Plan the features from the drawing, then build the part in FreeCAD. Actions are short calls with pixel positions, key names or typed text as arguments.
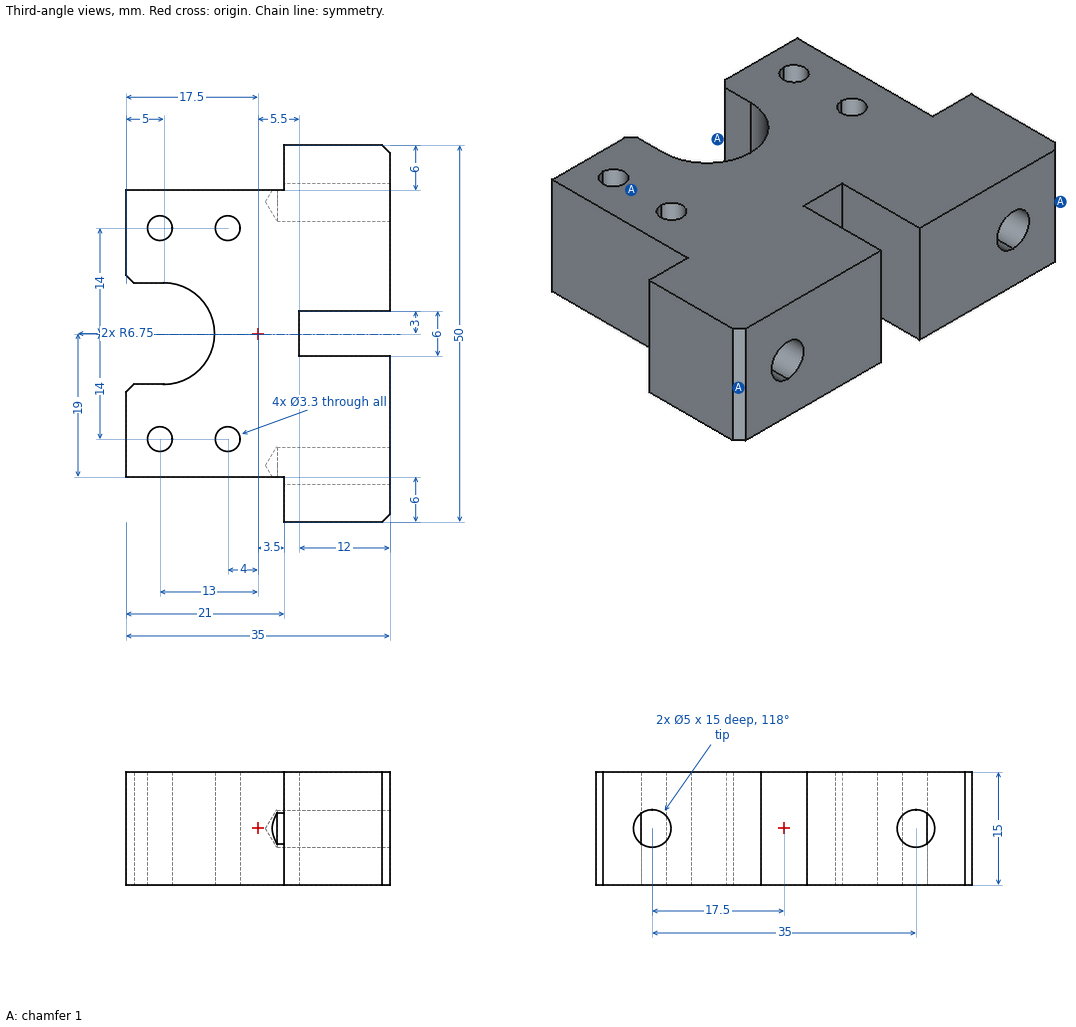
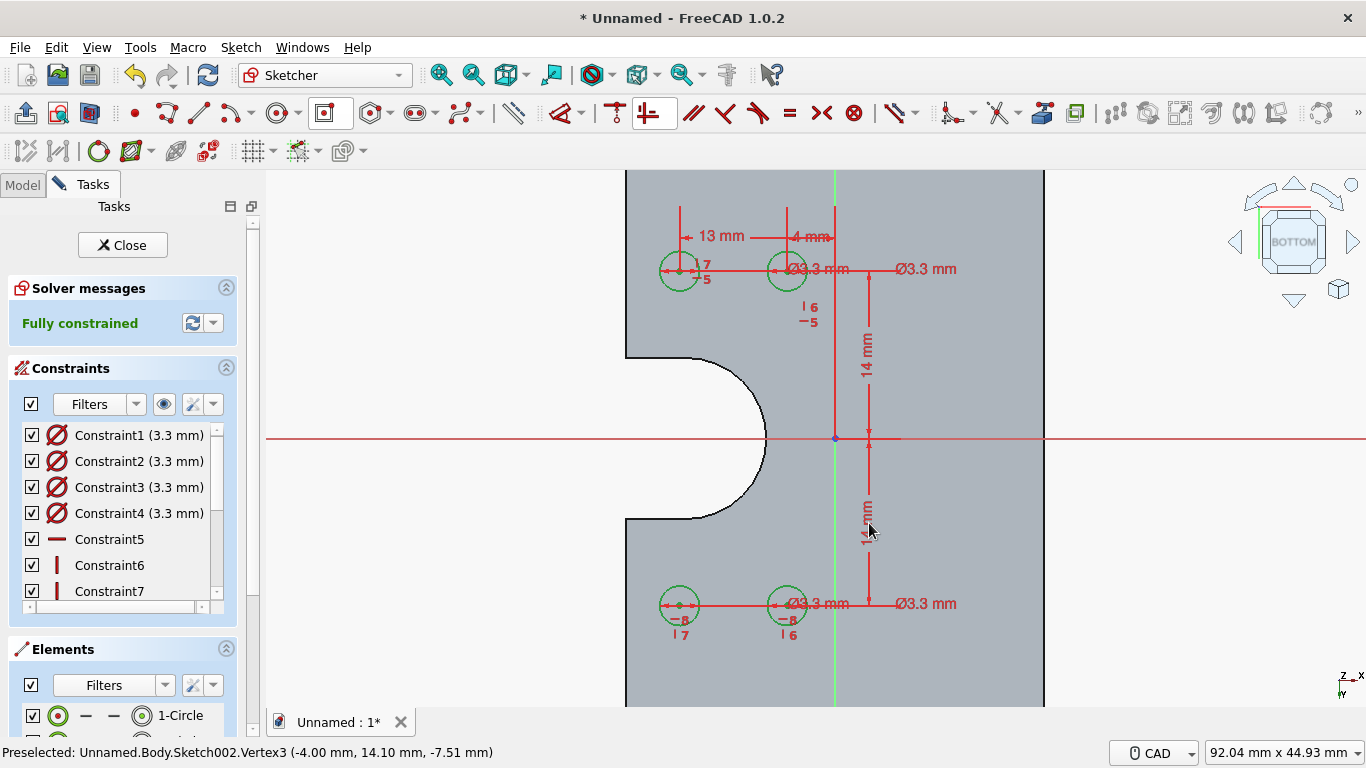
click(123, 245)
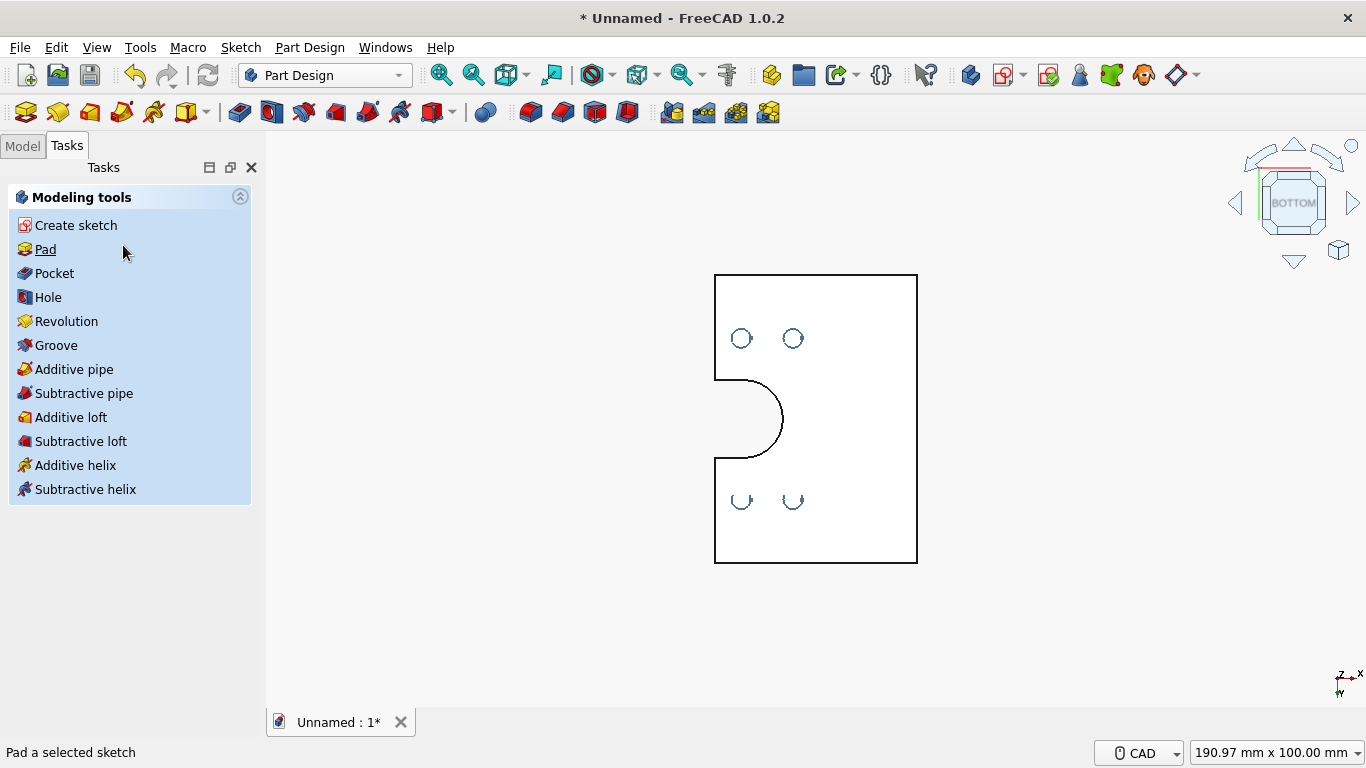
click(272, 112)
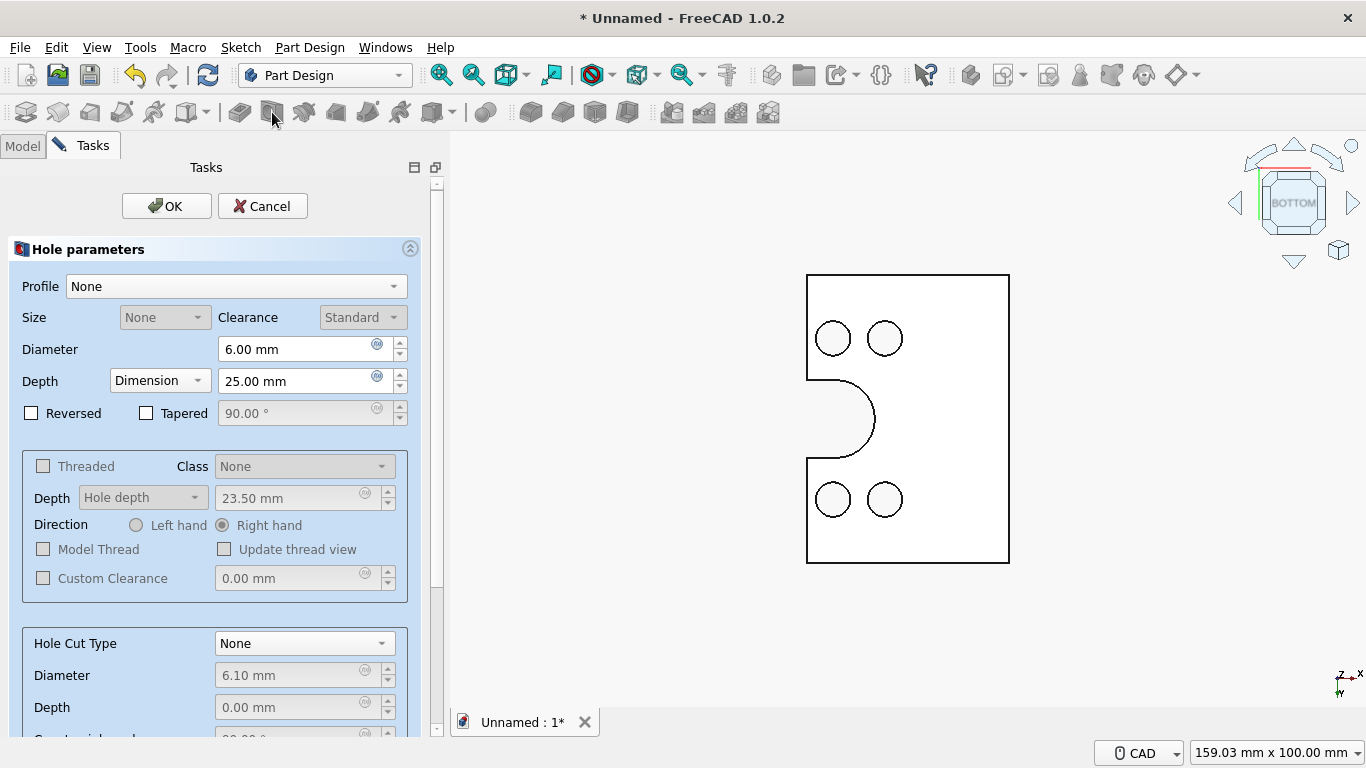
triple_click(305, 349)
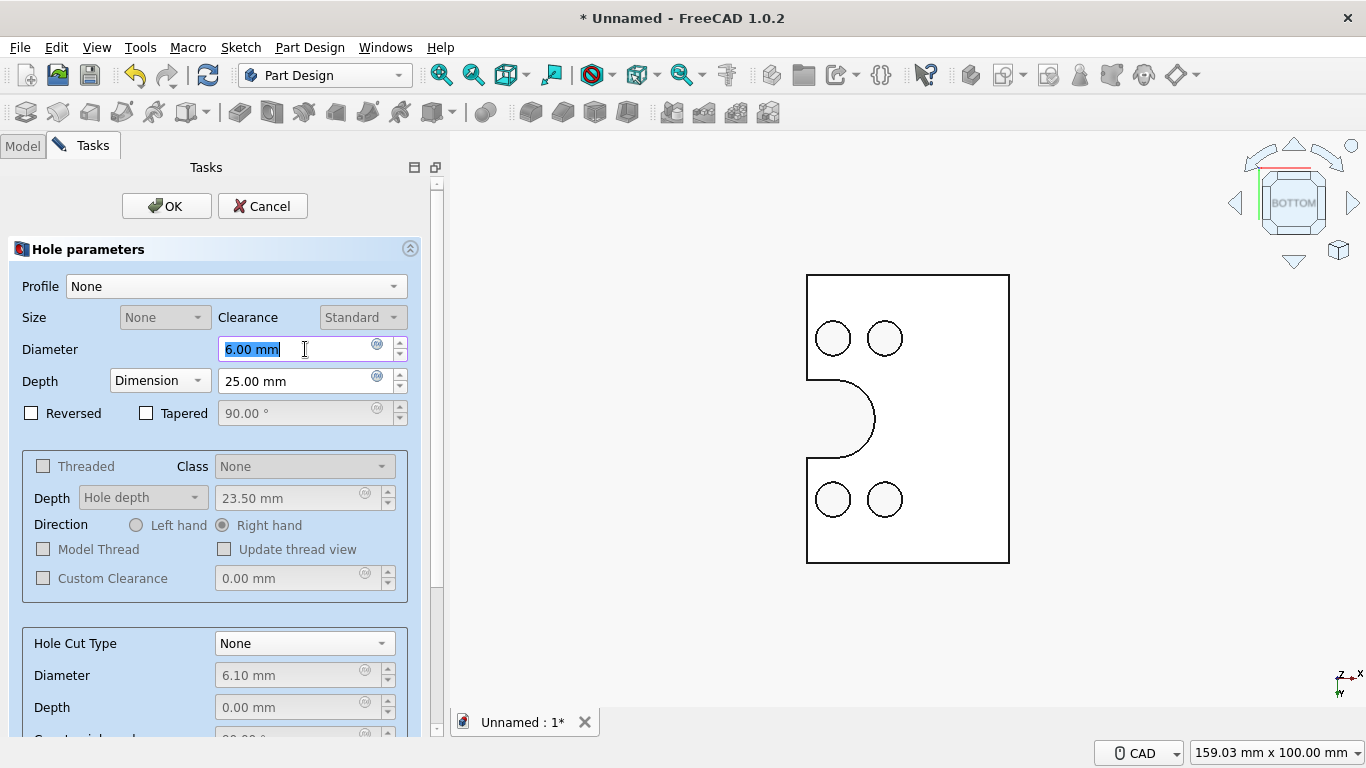
text(3.3)
key(Tab)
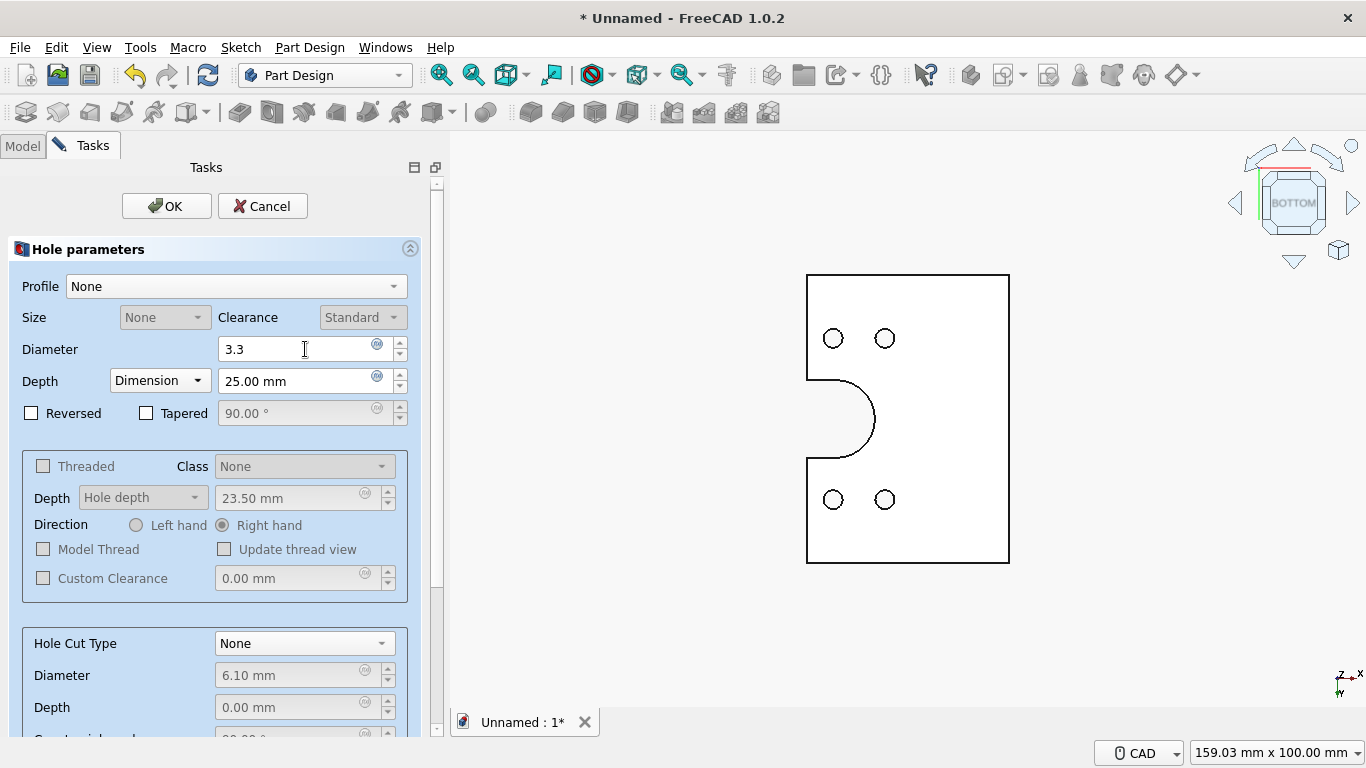
click(161, 380)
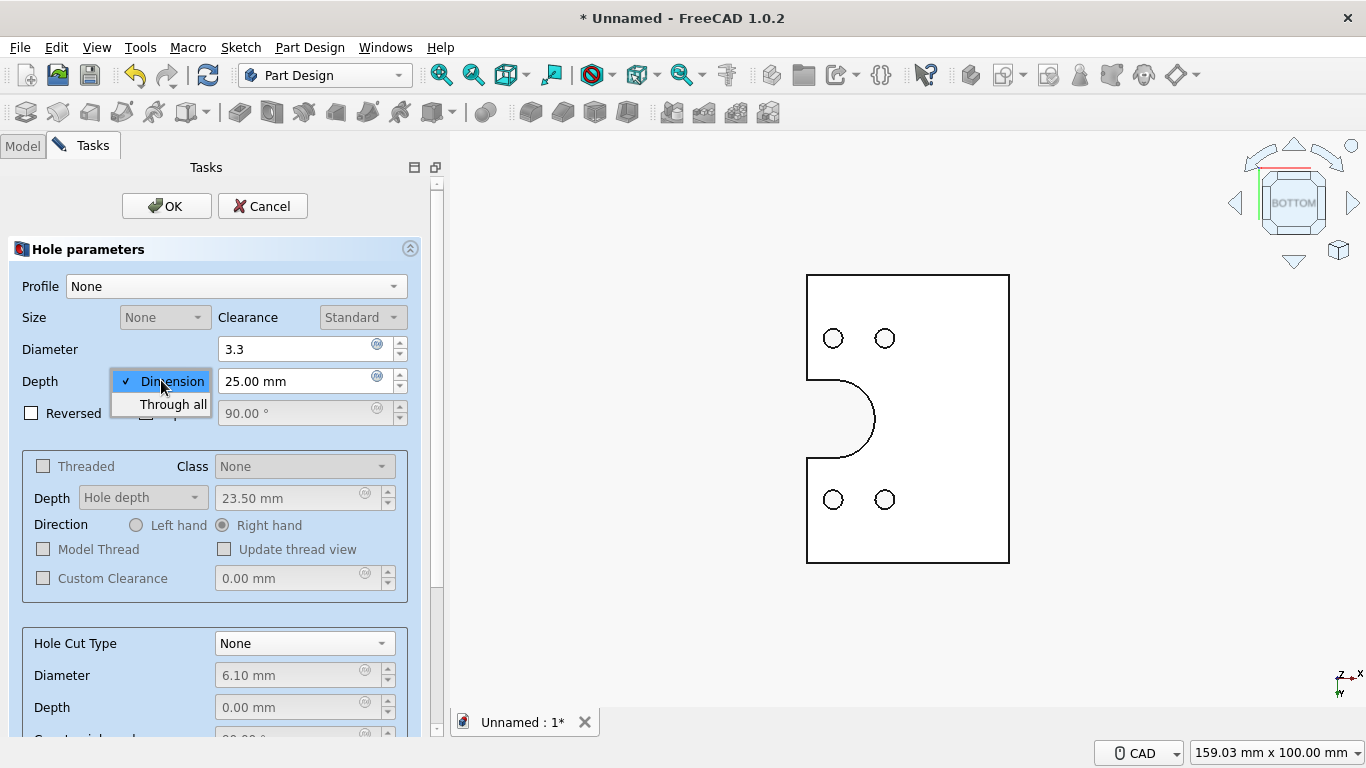
click(160, 404)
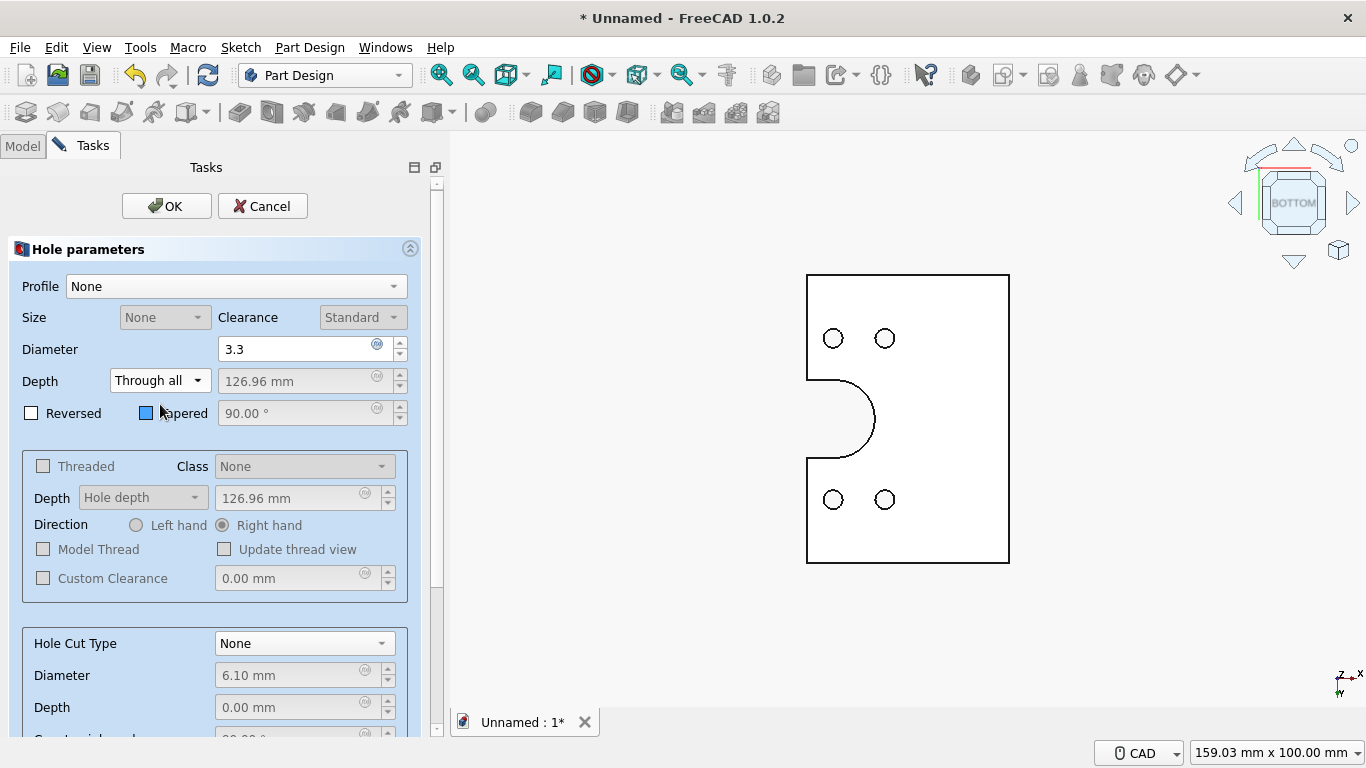
click(167, 206)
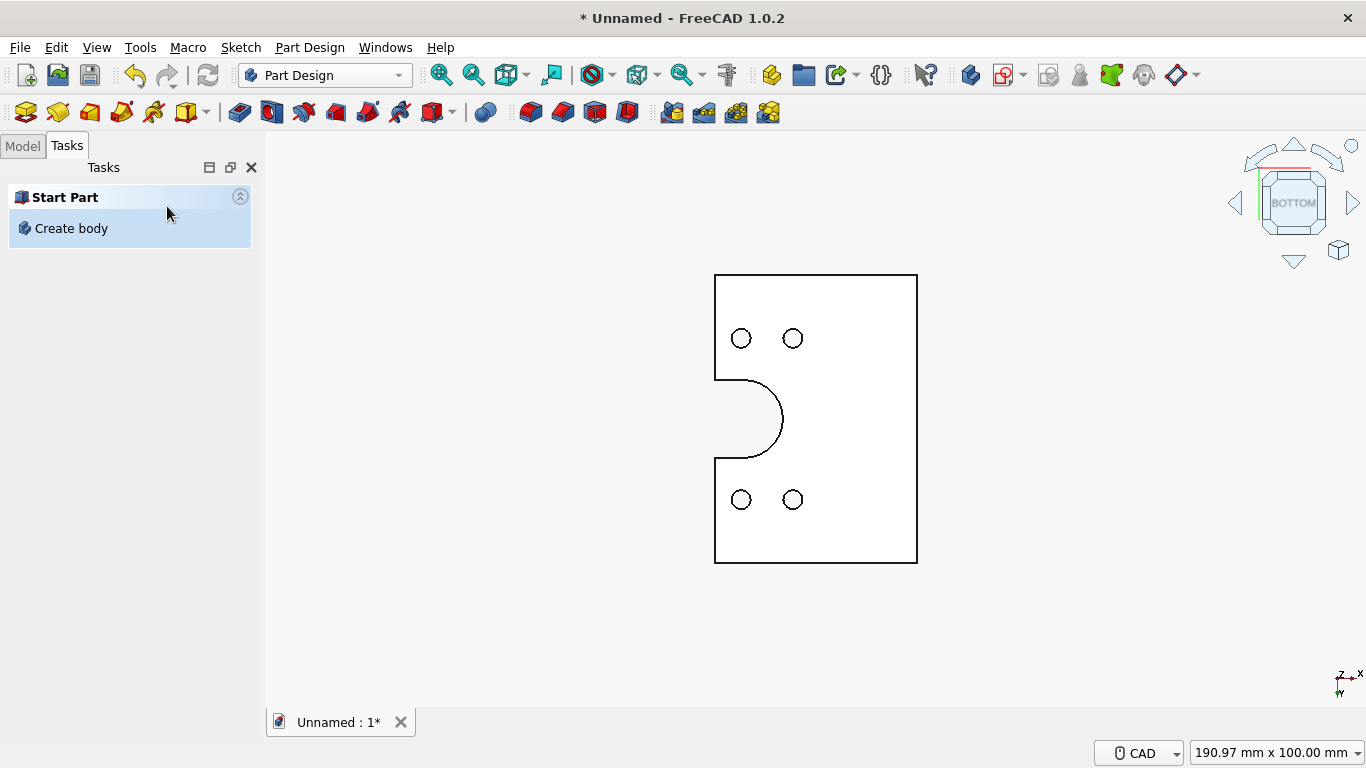
key(0)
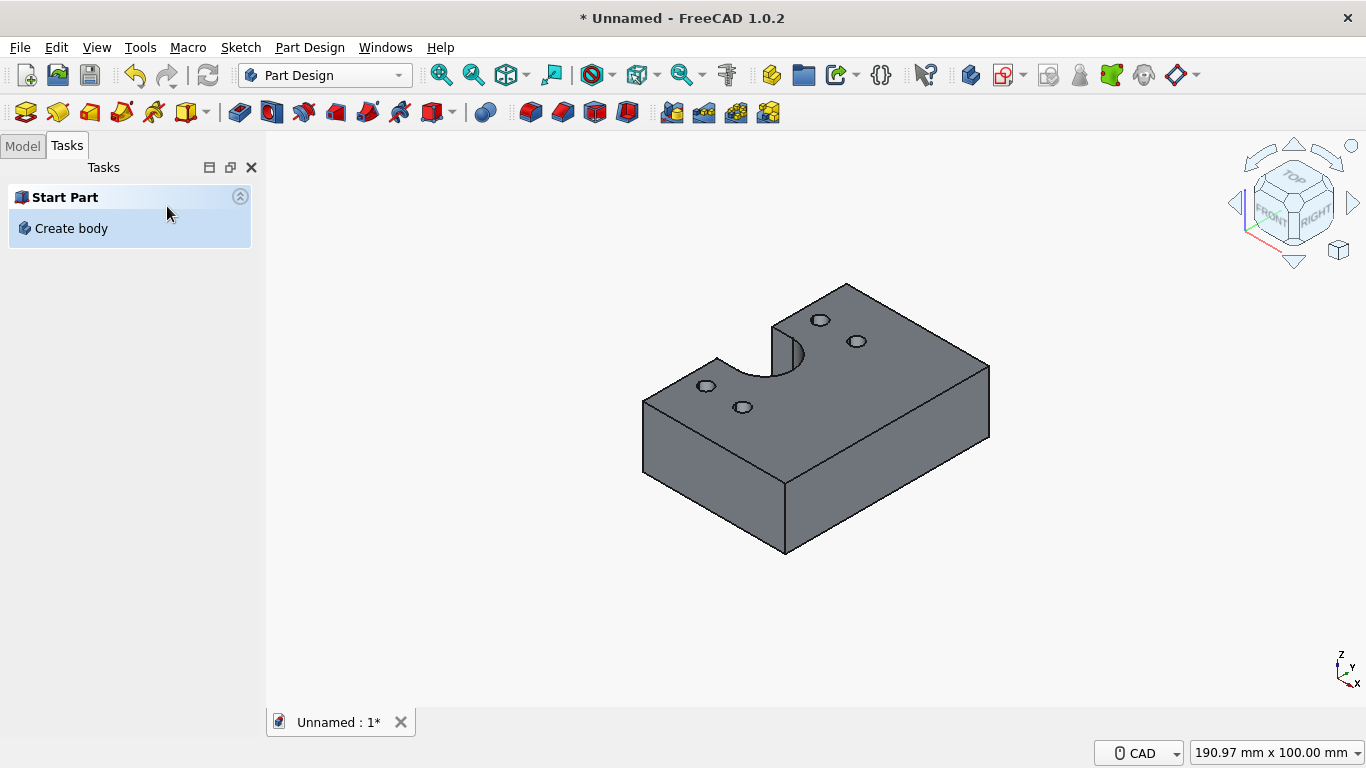
click(785, 518)